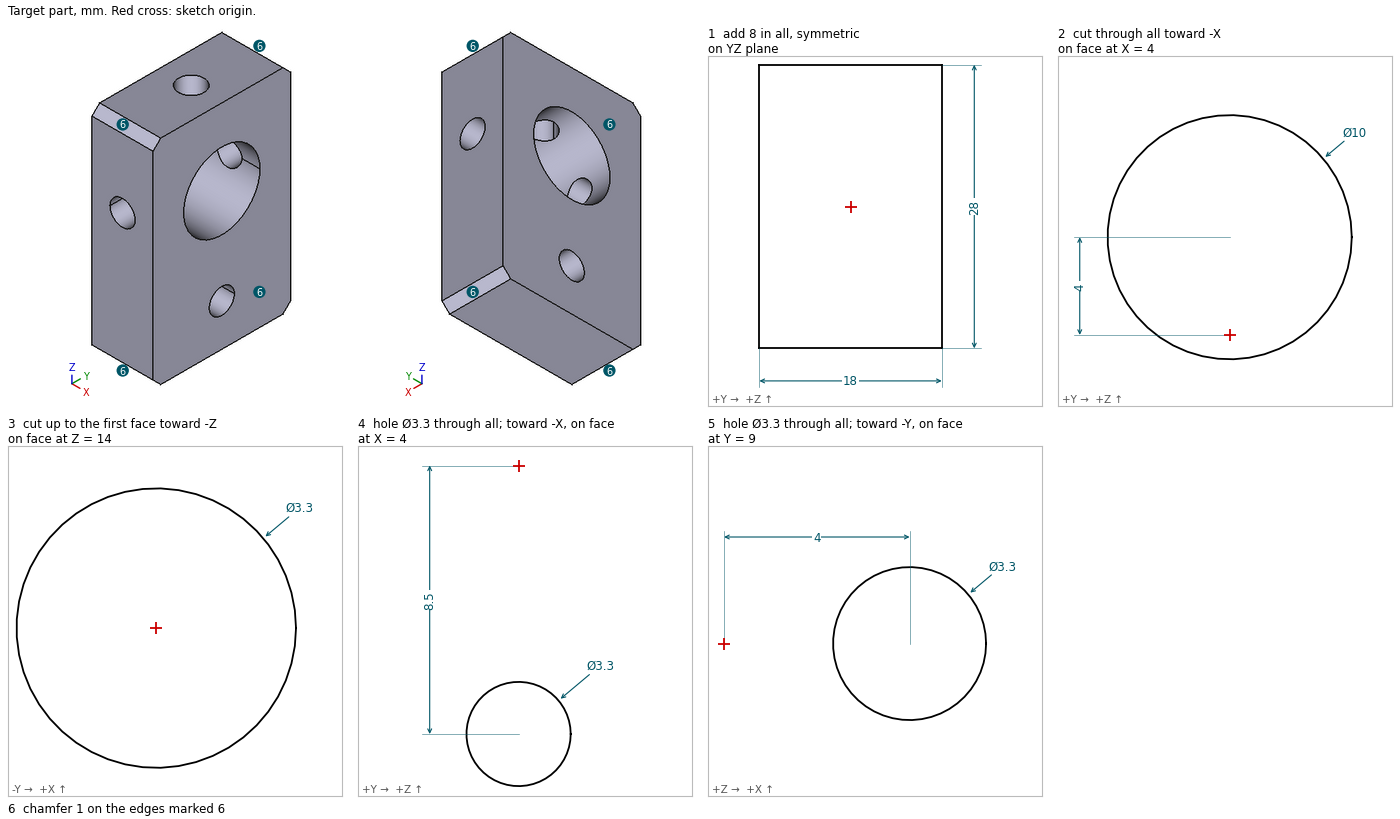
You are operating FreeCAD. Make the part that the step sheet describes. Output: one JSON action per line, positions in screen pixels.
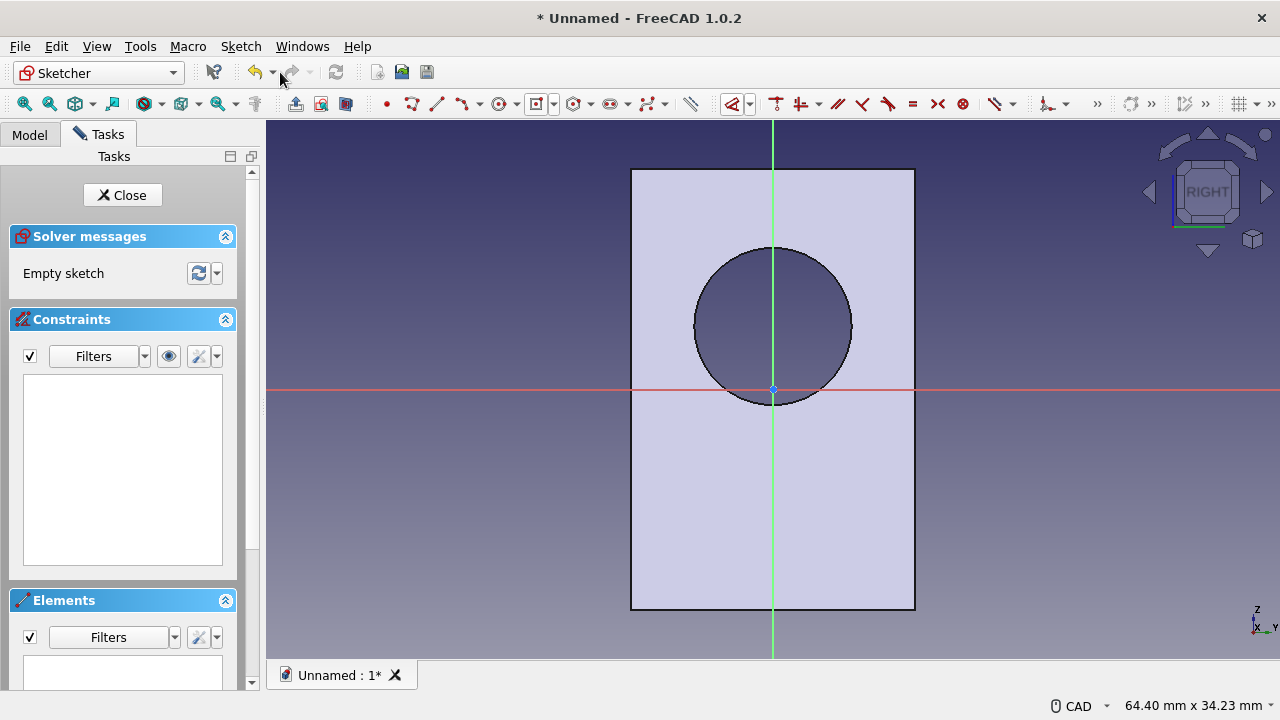
{"action": "scroll", "coordinate": [787, 550], "scroll_direction": "up", "scroll_amount": 9}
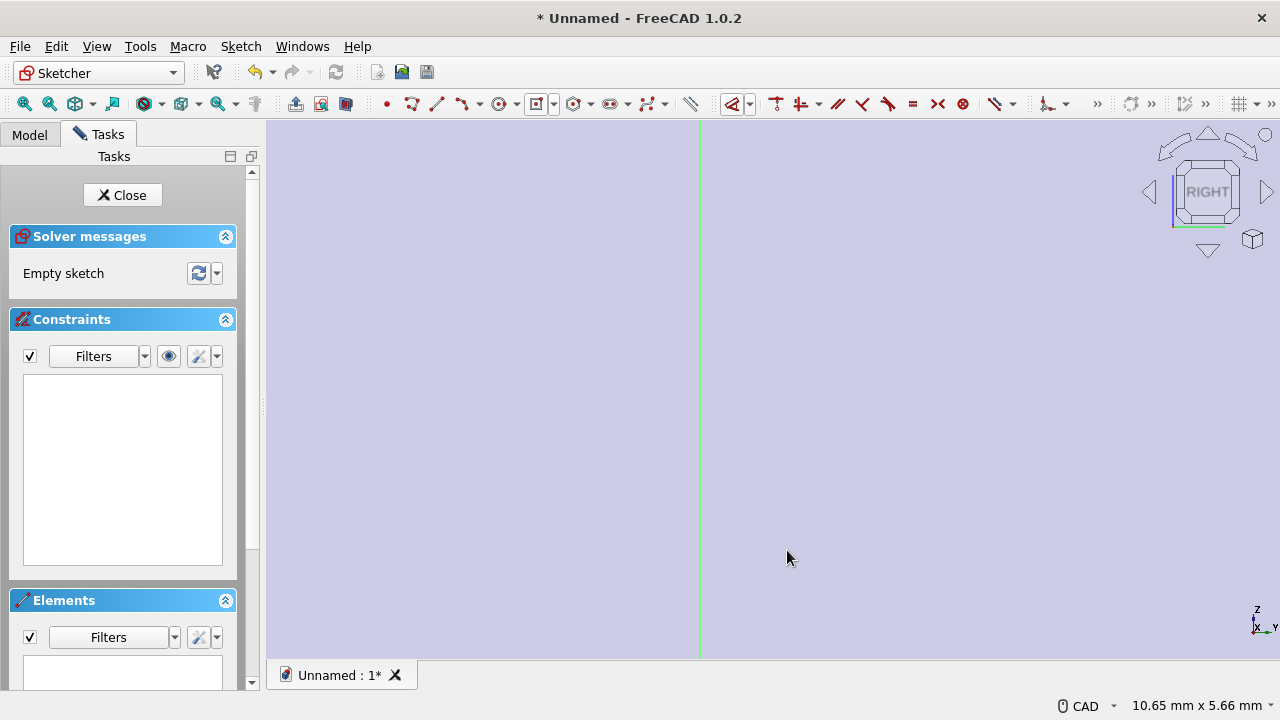
{"action": "left_click", "coordinate": [498, 104]}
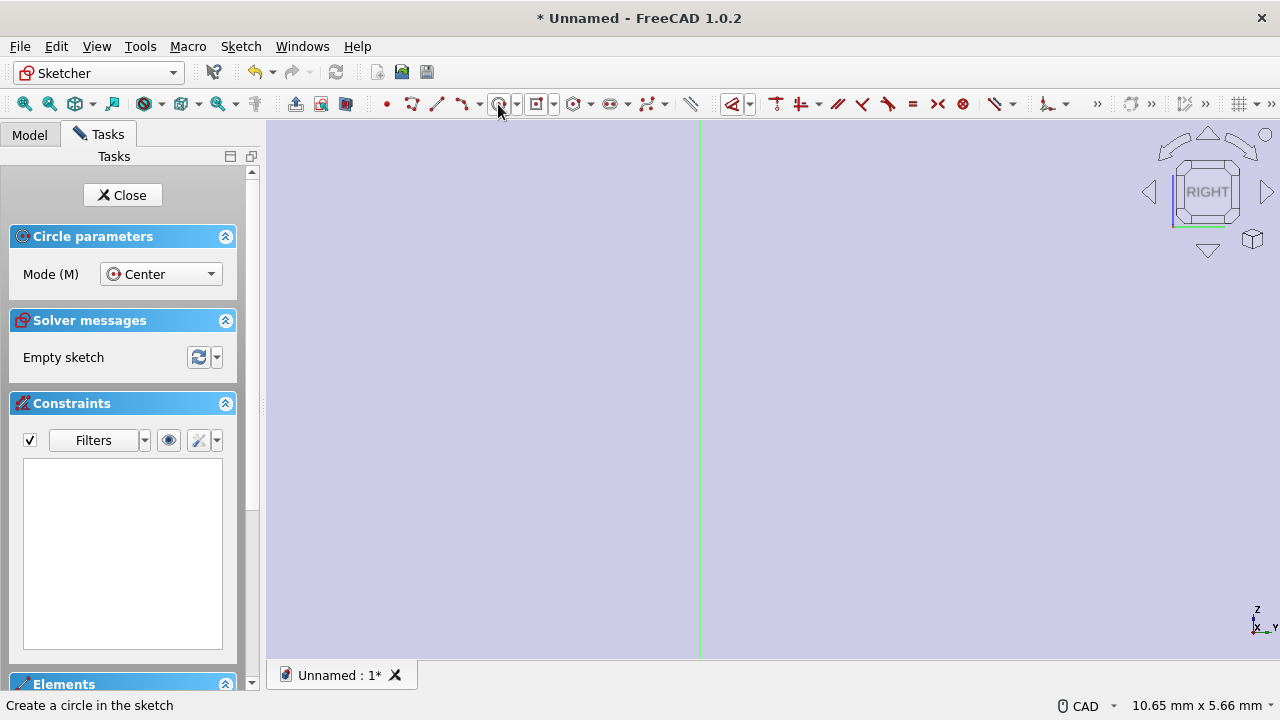
{"action": "left_click", "coordinate": [700, 385]}
{"action": "left_click", "coordinate": [811, 273]}
{"action": "key", "text": "Escape"}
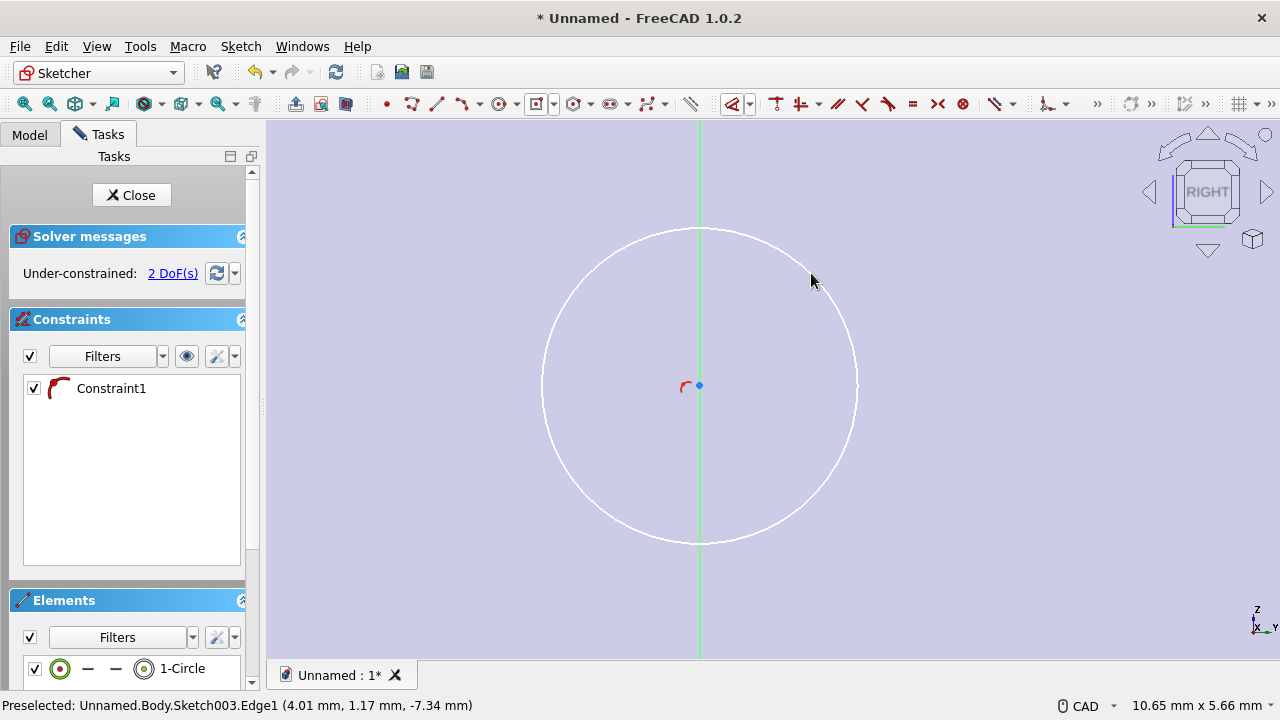
{"action": "left_click", "coordinate": [811, 274]}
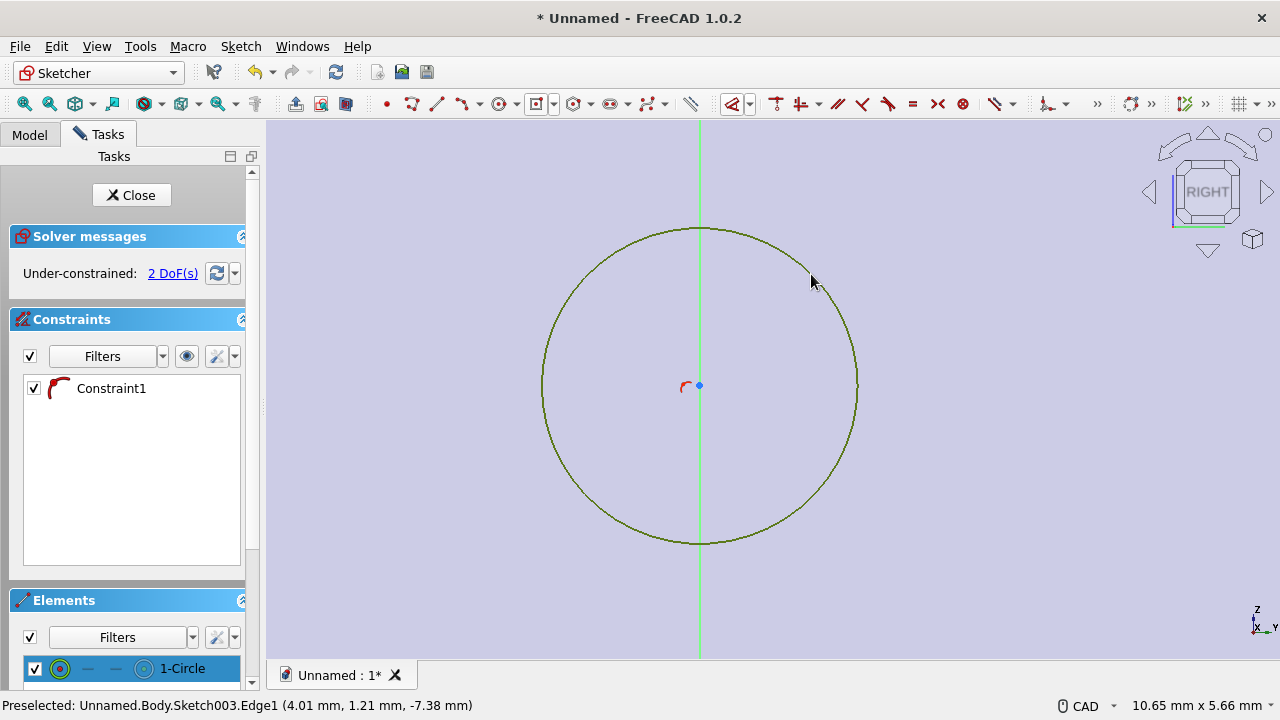
{"action": "key", "text": "k o"}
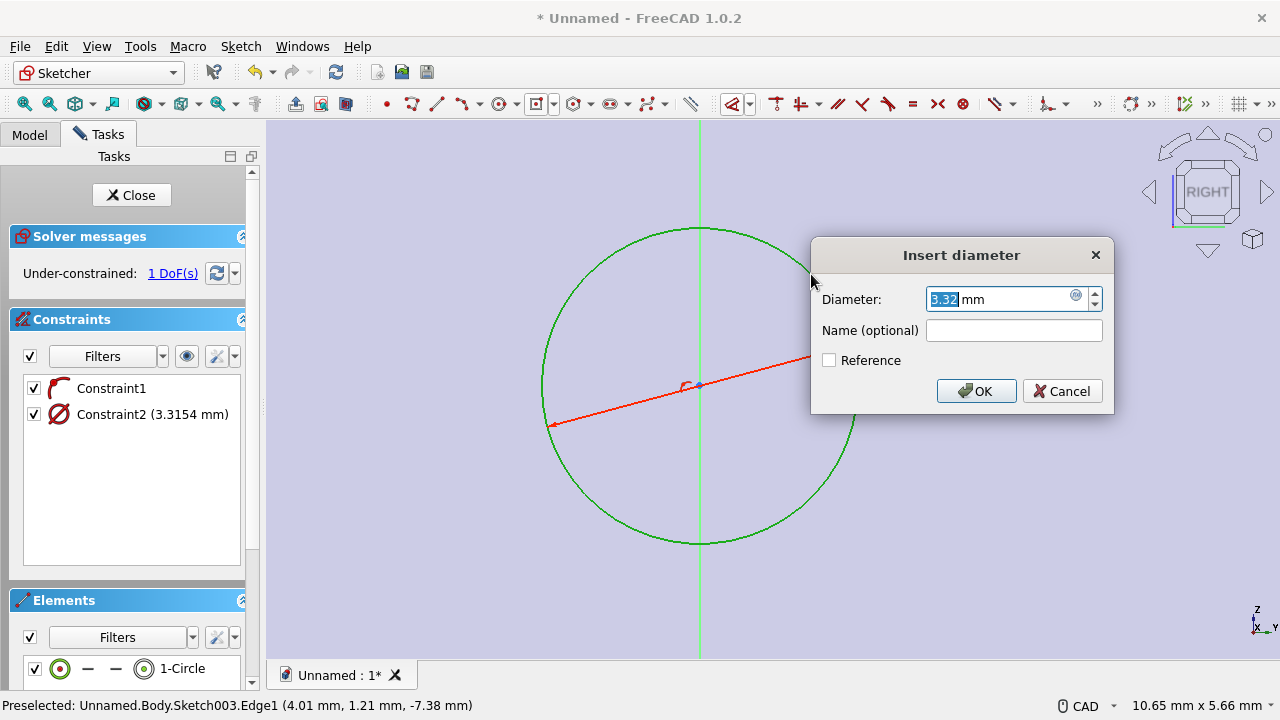
{"action": "type", "text": "3.3"}
{"action": "key", "text": "Return"}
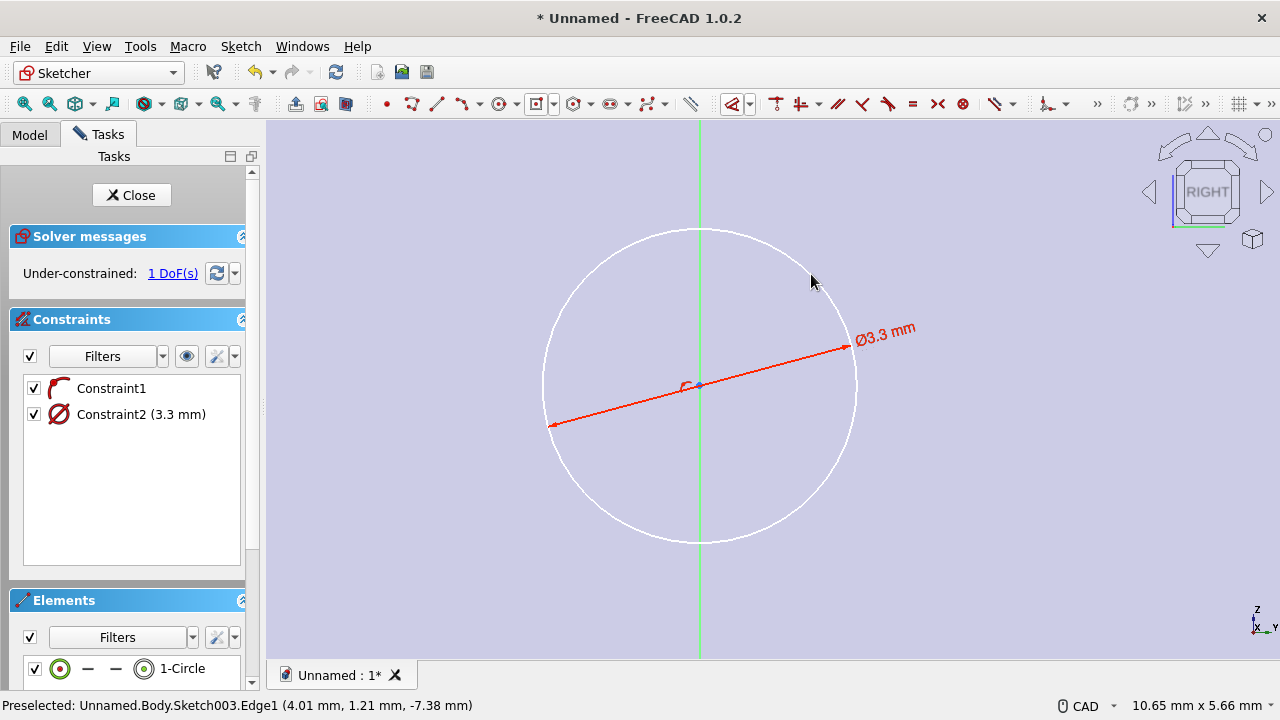
{"action": "left_click", "coordinate": [700, 386]}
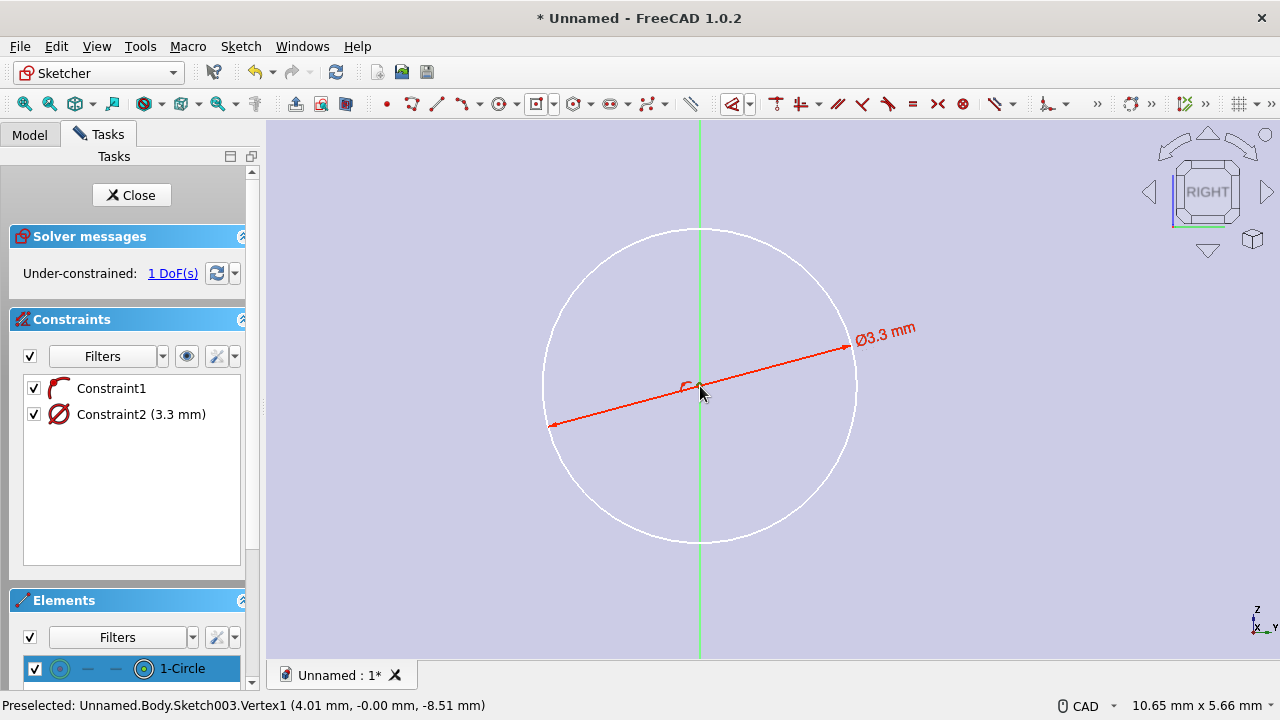
{"action": "left_click", "coordinate": [750, 104]}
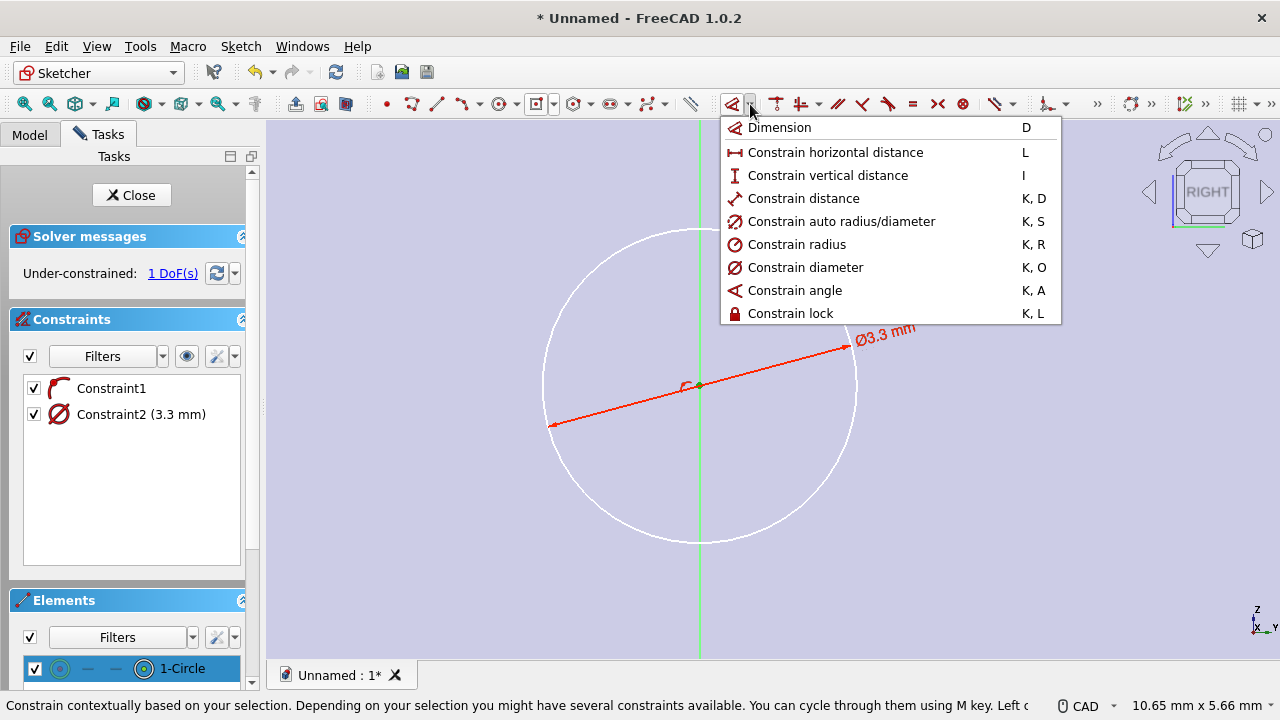
{"action": "left_click", "coordinate": [891, 176]}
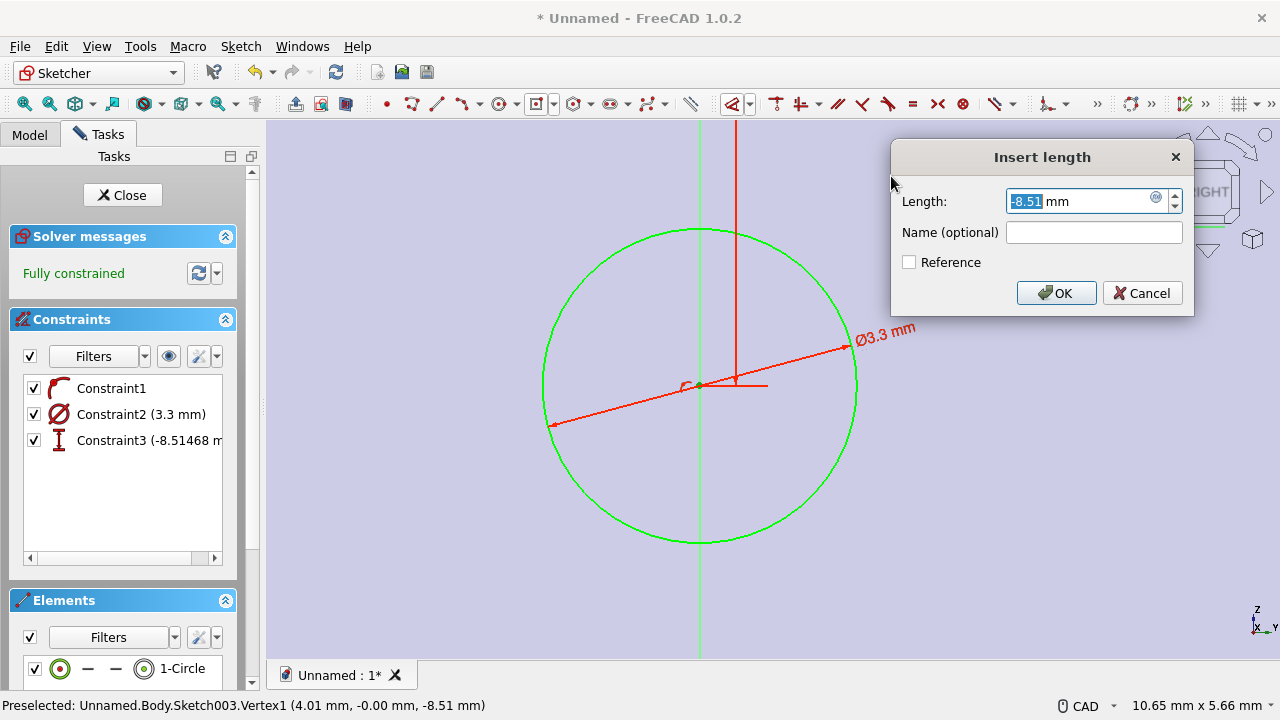
{"action": "type", "text": "-8.5"}
{"action": "key", "text": "Return"}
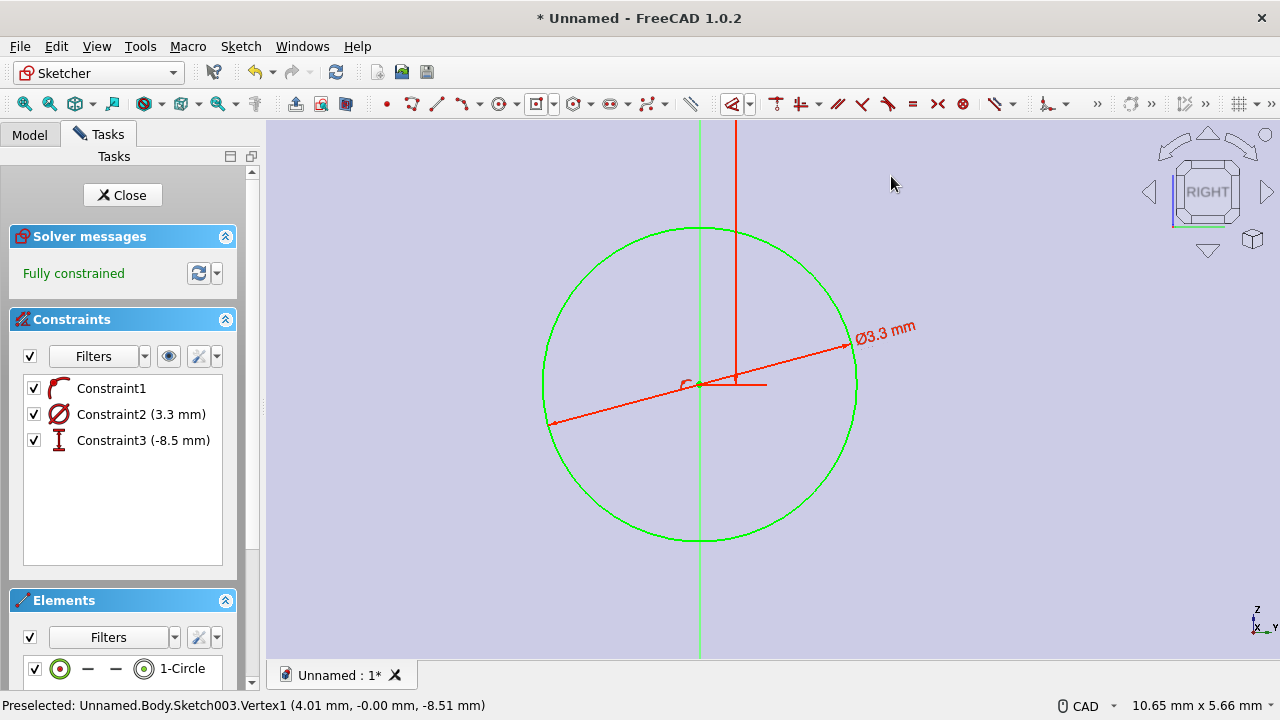
{"action": "left_click", "coordinate": [123, 195]}